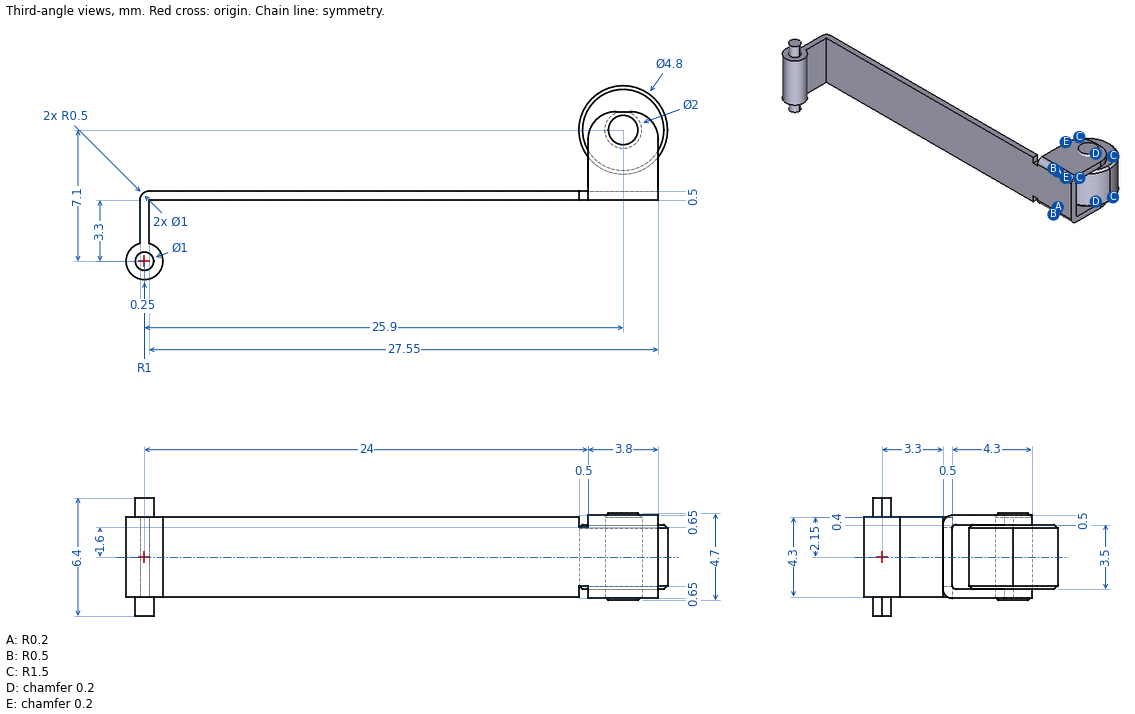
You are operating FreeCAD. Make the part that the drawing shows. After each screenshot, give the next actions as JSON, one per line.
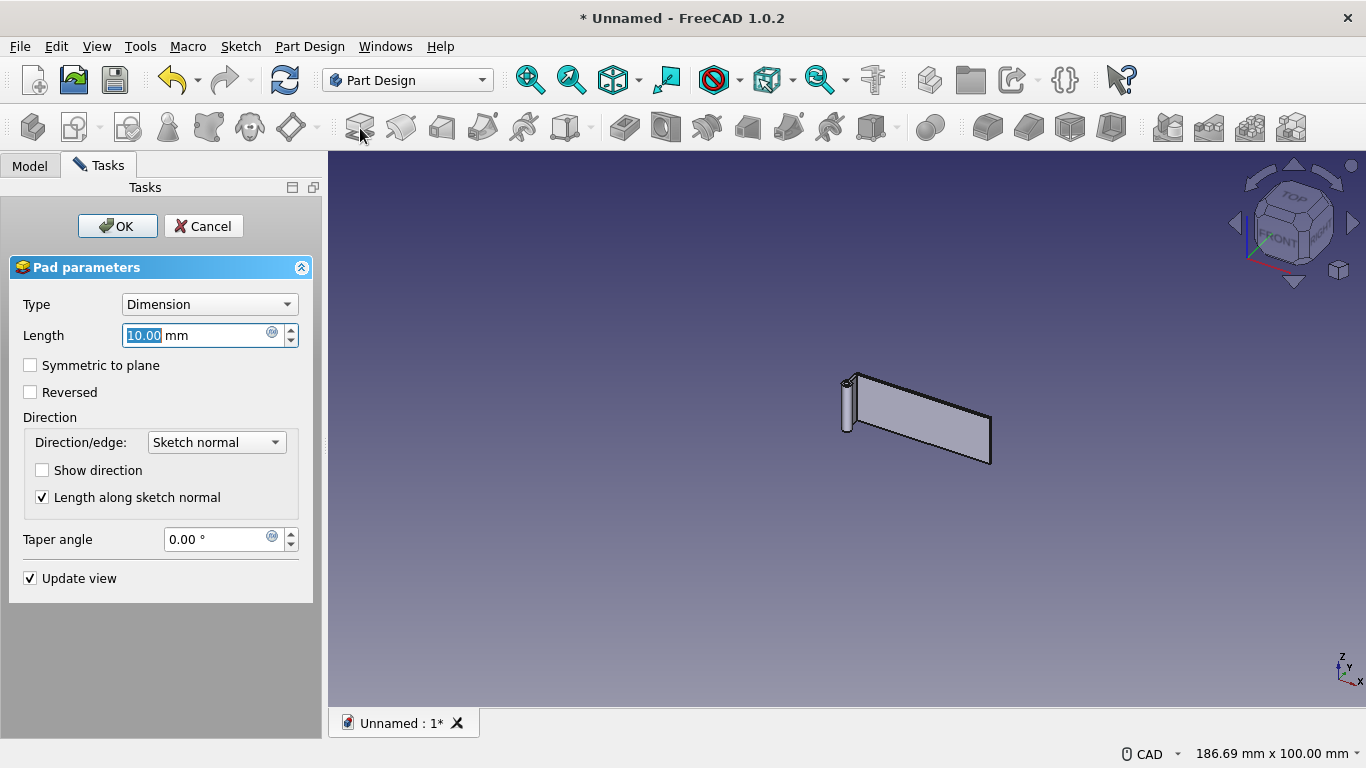
{"action": "type", "text": "4.3"}
{"action": "key", "text": "Tab"}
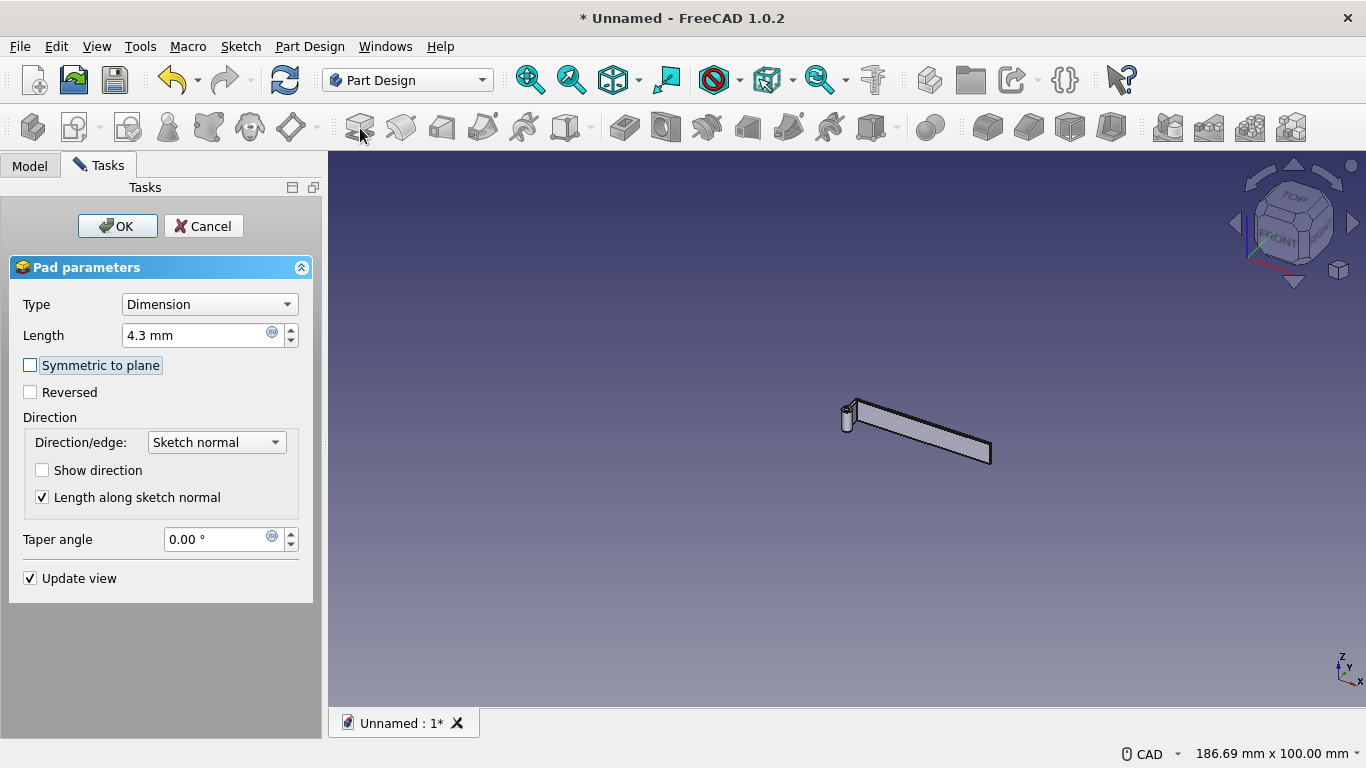
{"action": "left_click", "coordinate": [31, 365]}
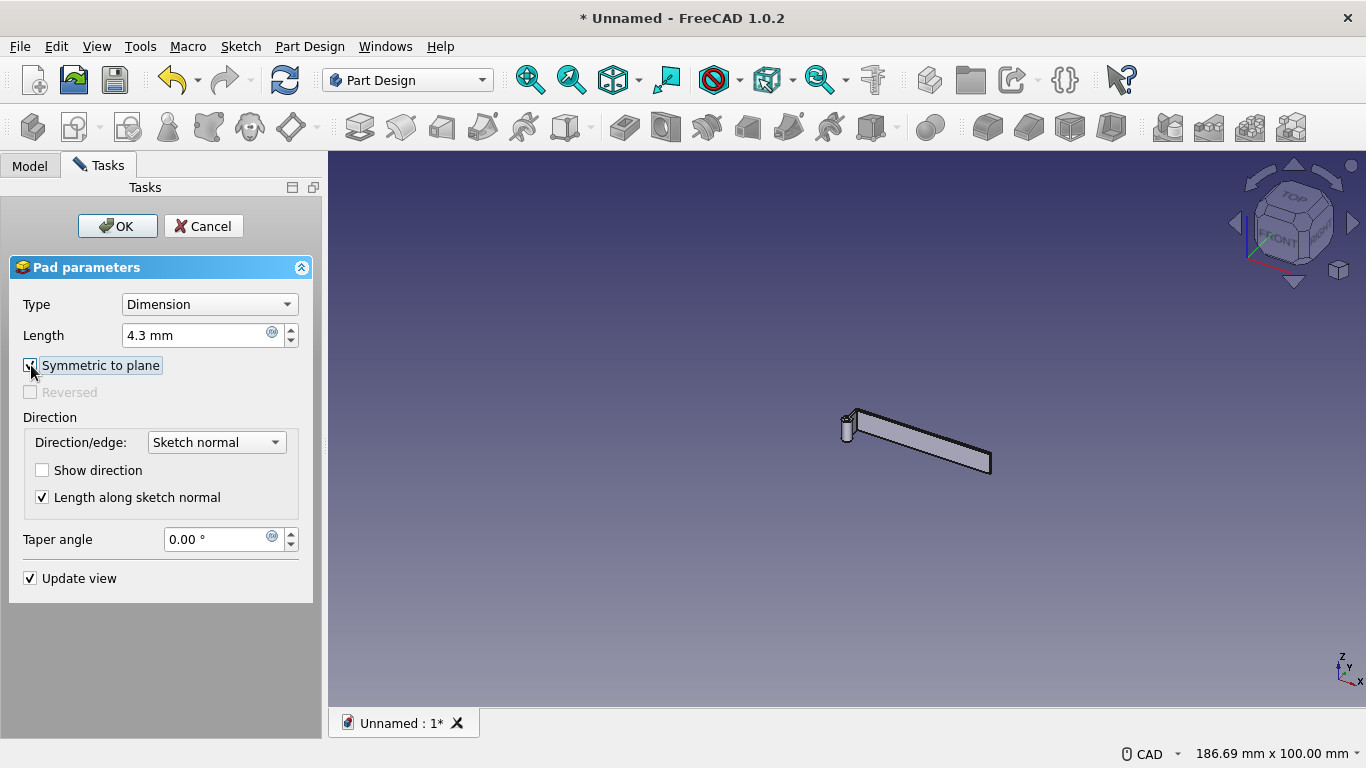
{"action": "left_click", "coordinate": [118, 226]}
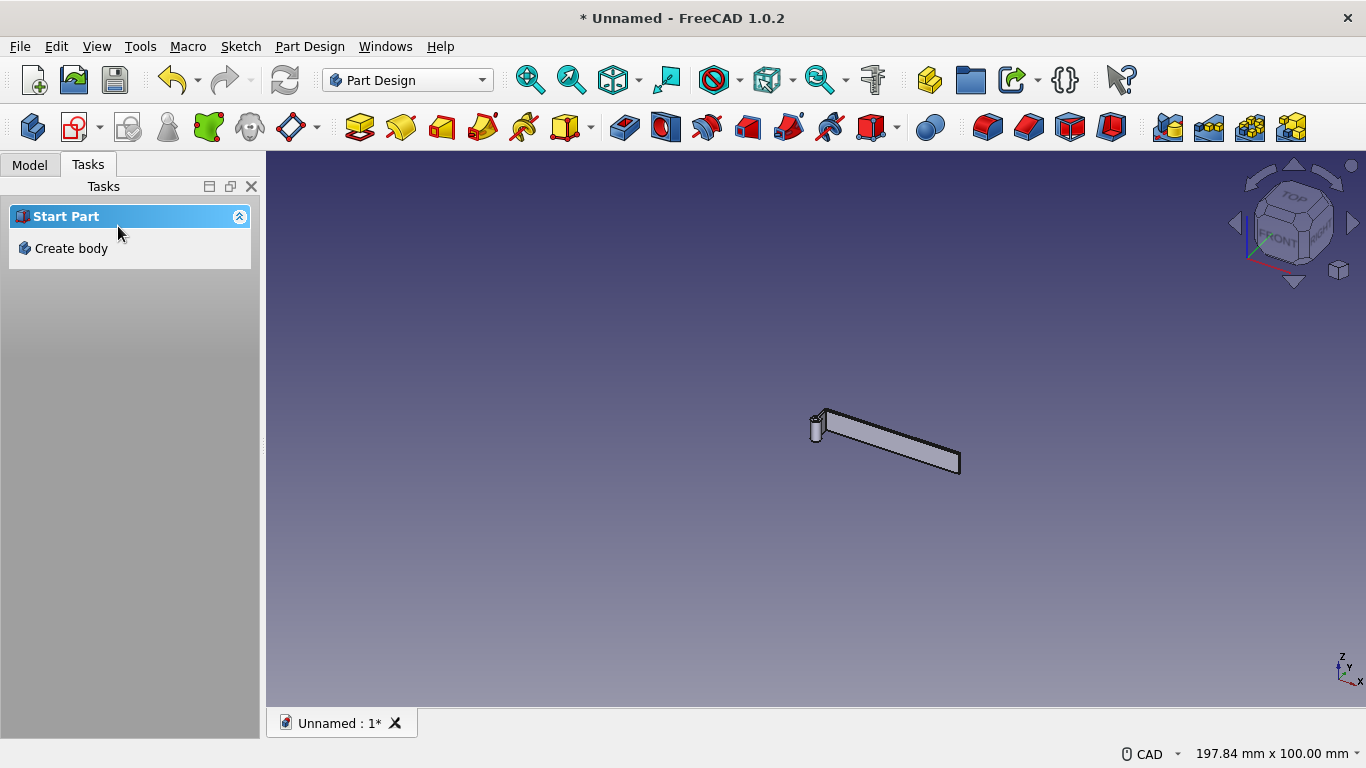
{"action": "left_click", "coordinate": [531, 80]}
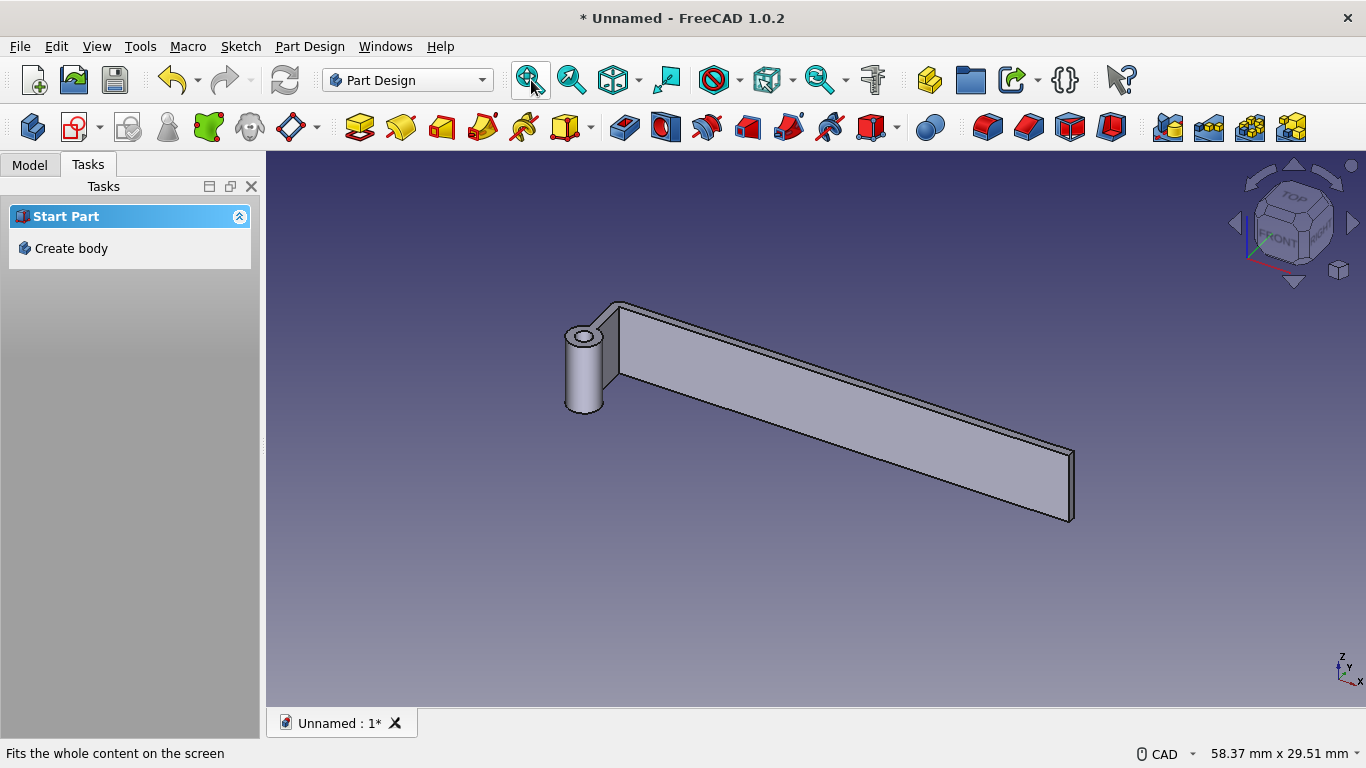
{"action": "left_click", "coordinate": [74, 128]}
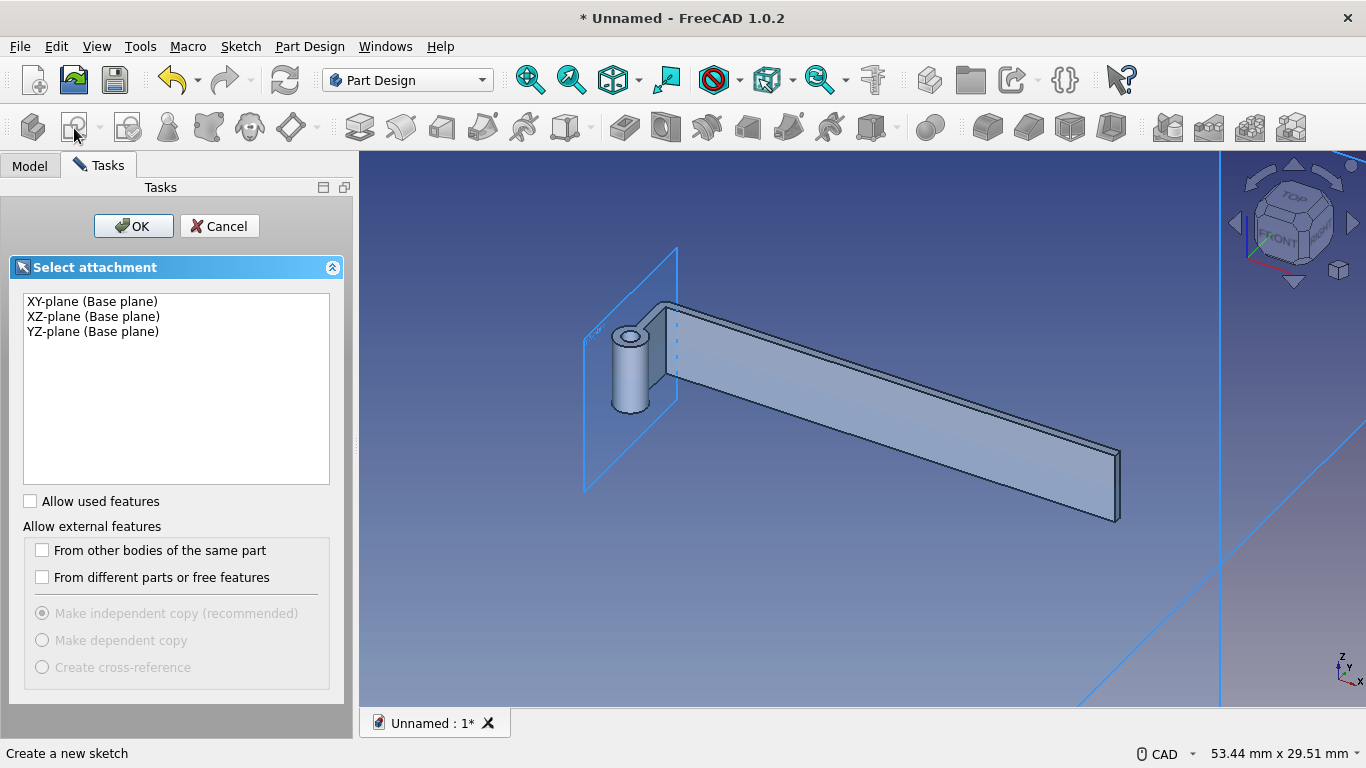
{"action": "left_click", "coordinate": [84, 302]}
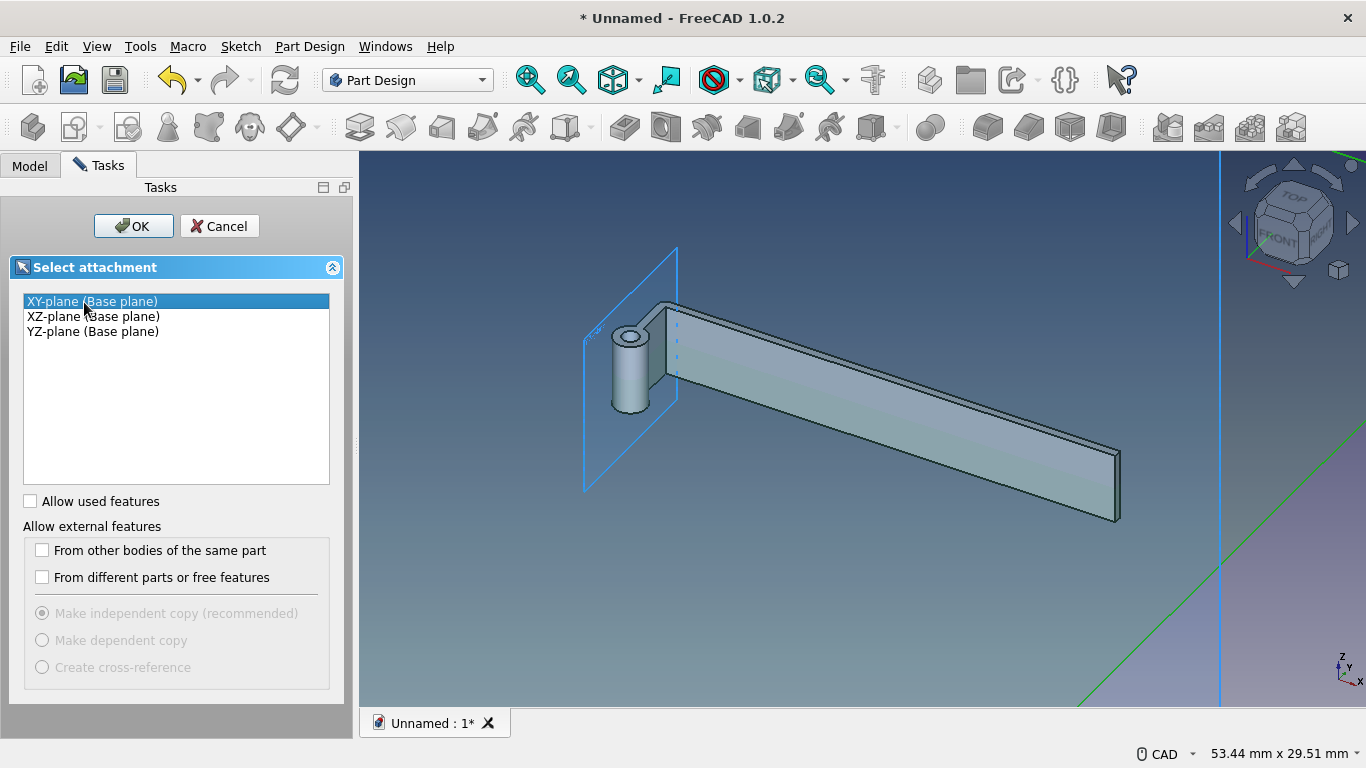
{"action": "left_click", "coordinate": [134, 226]}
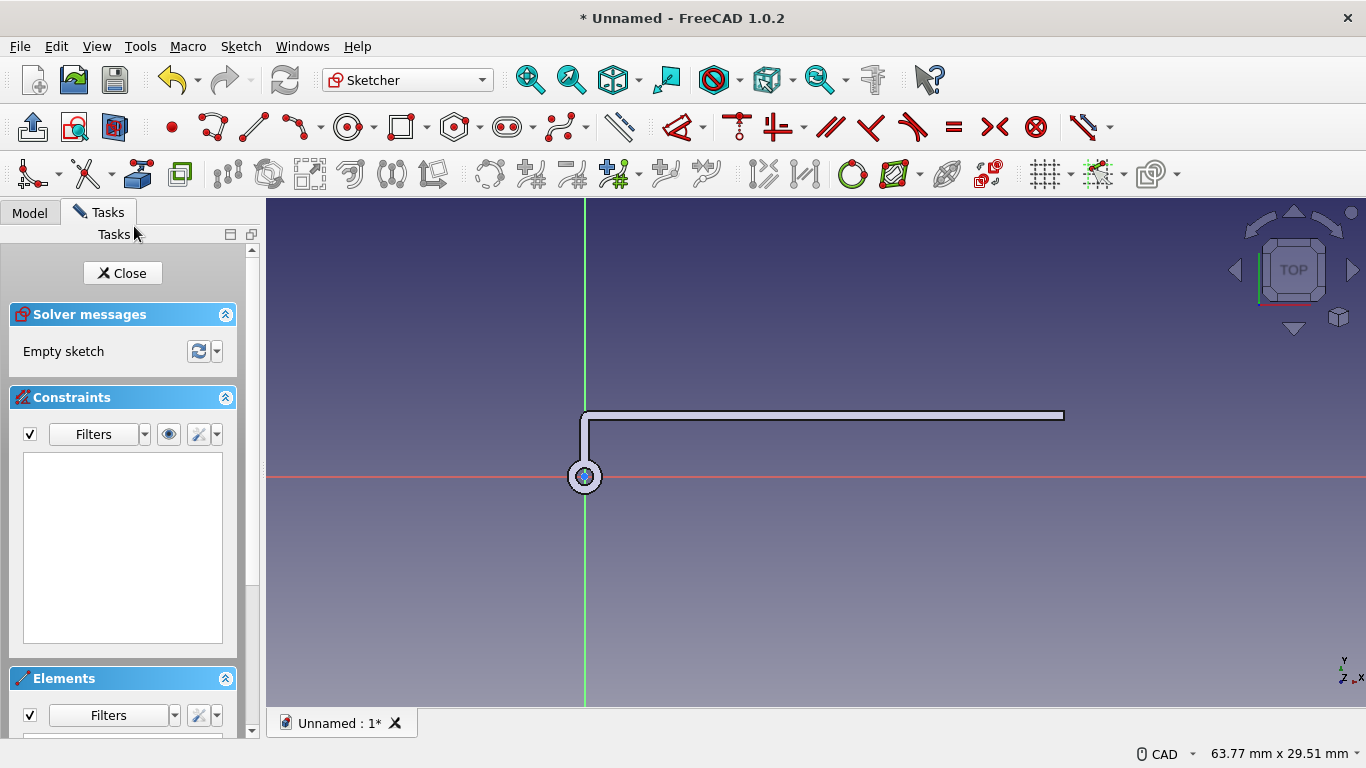
{"action": "key", "text": "q s"}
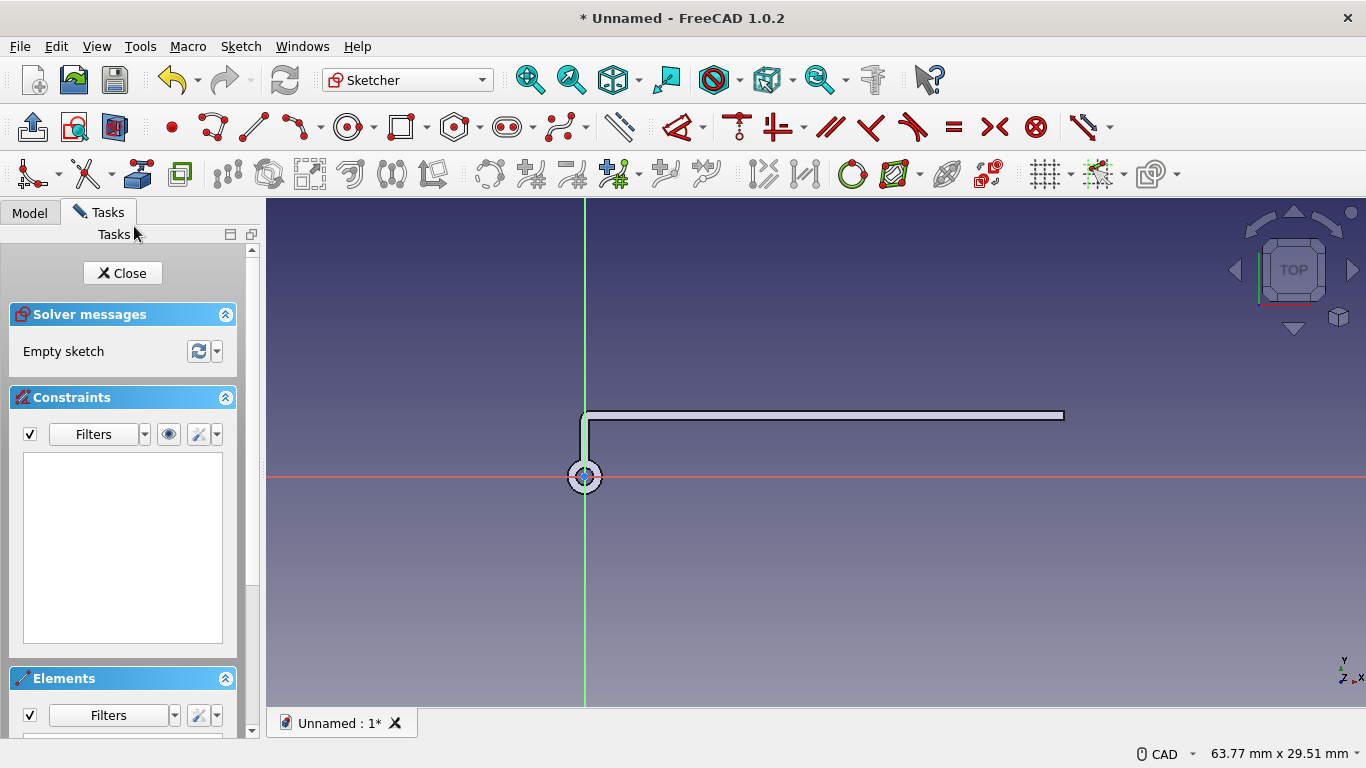
{"action": "scroll", "coordinate": [576, 478], "scroll_direction": "up", "scroll_amount": 15}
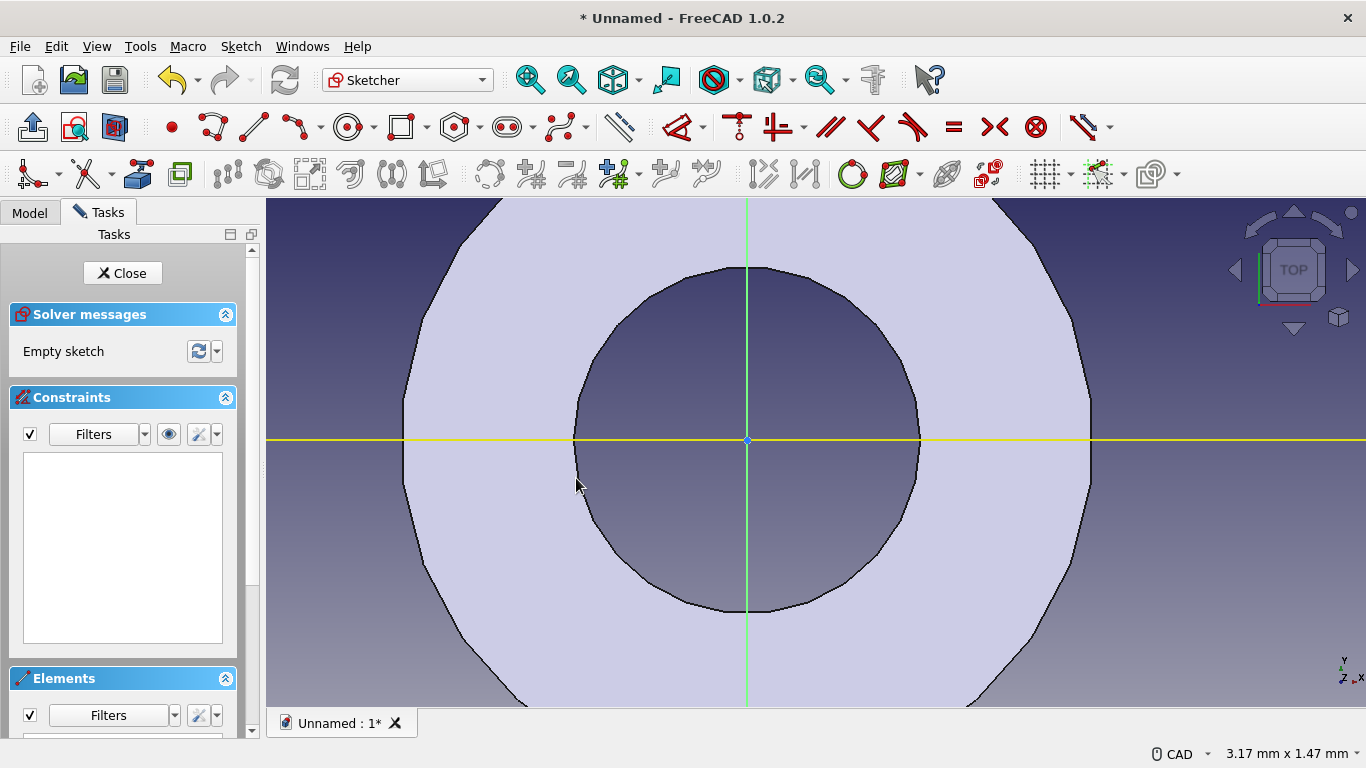
{"action": "key", "text": "g c"}